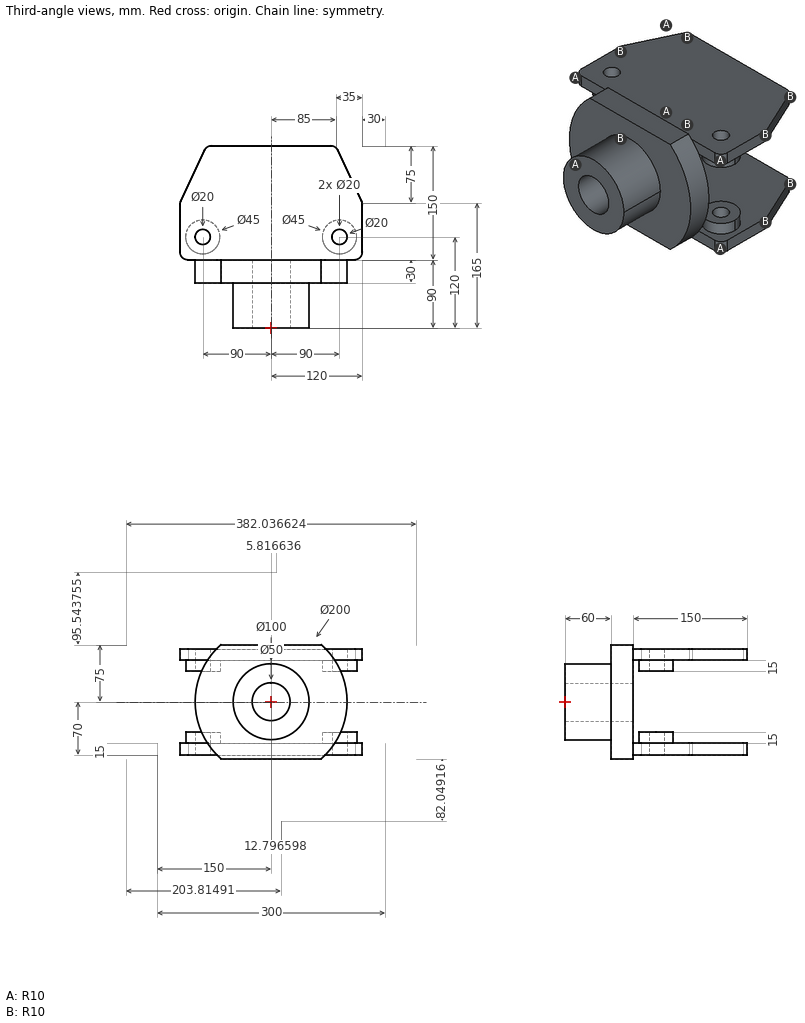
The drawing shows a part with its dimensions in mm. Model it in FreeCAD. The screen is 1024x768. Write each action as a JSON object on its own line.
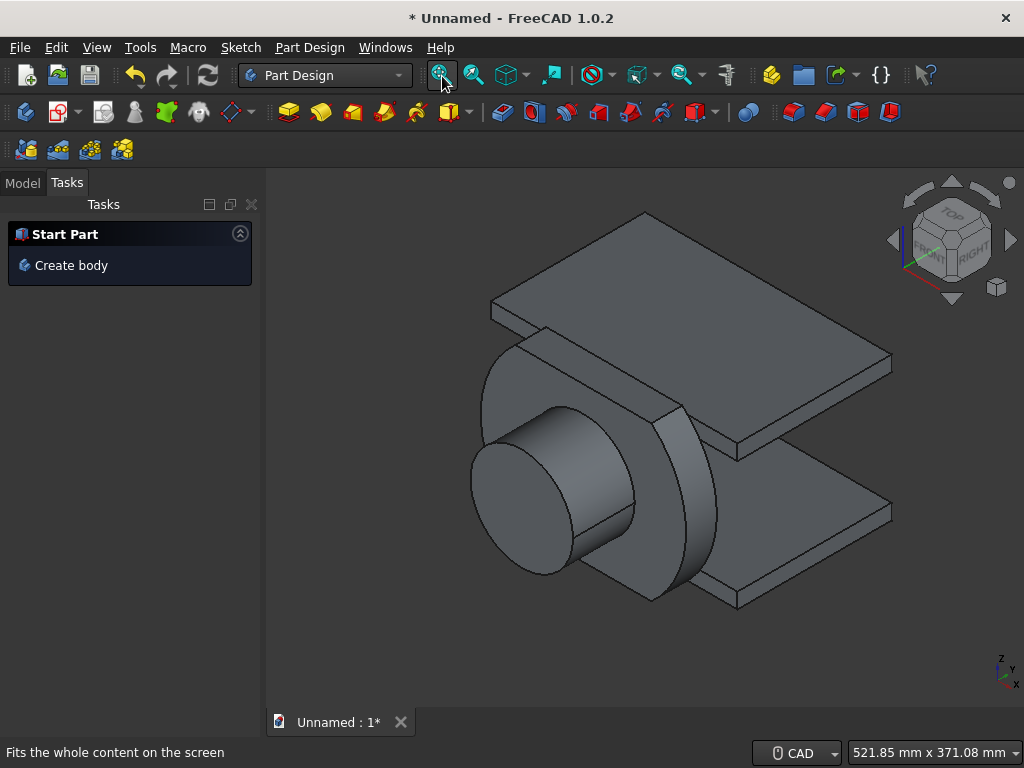
{"action": "left_click", "coordinate": [737, 600]}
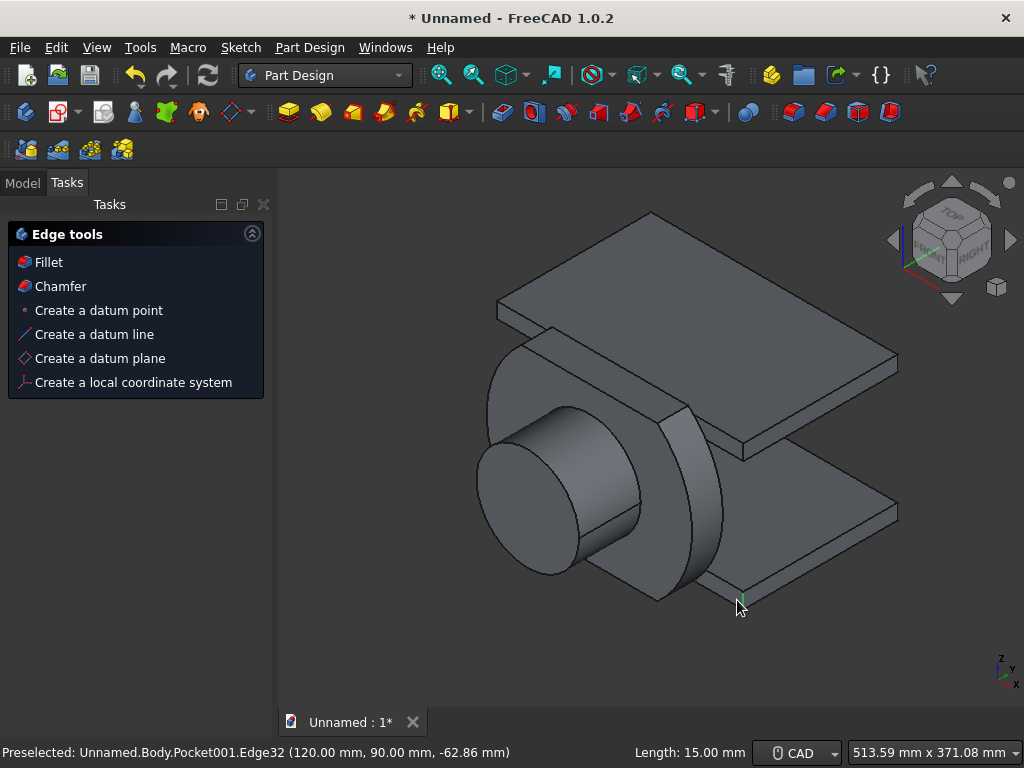
{"action": "left_click", "coordinate": [743, 451], "text": "ctrl"}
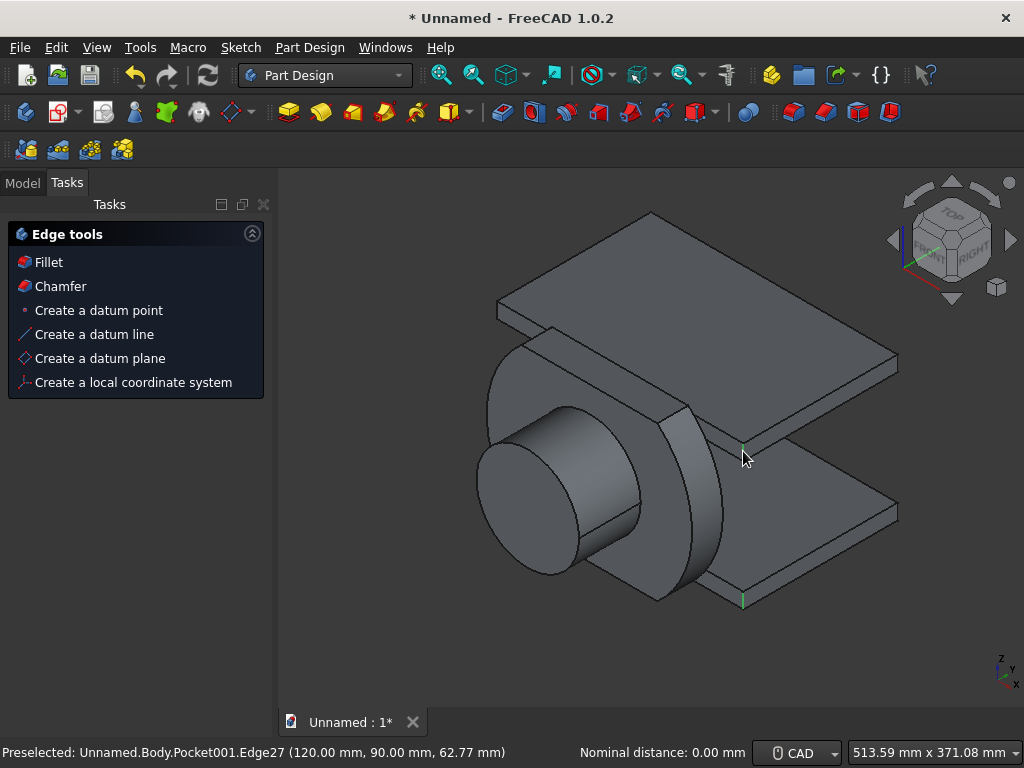
{"action": "scroll", "coordinate": [651, 368], "scroll_direction": "up", "scroll_amount": 4}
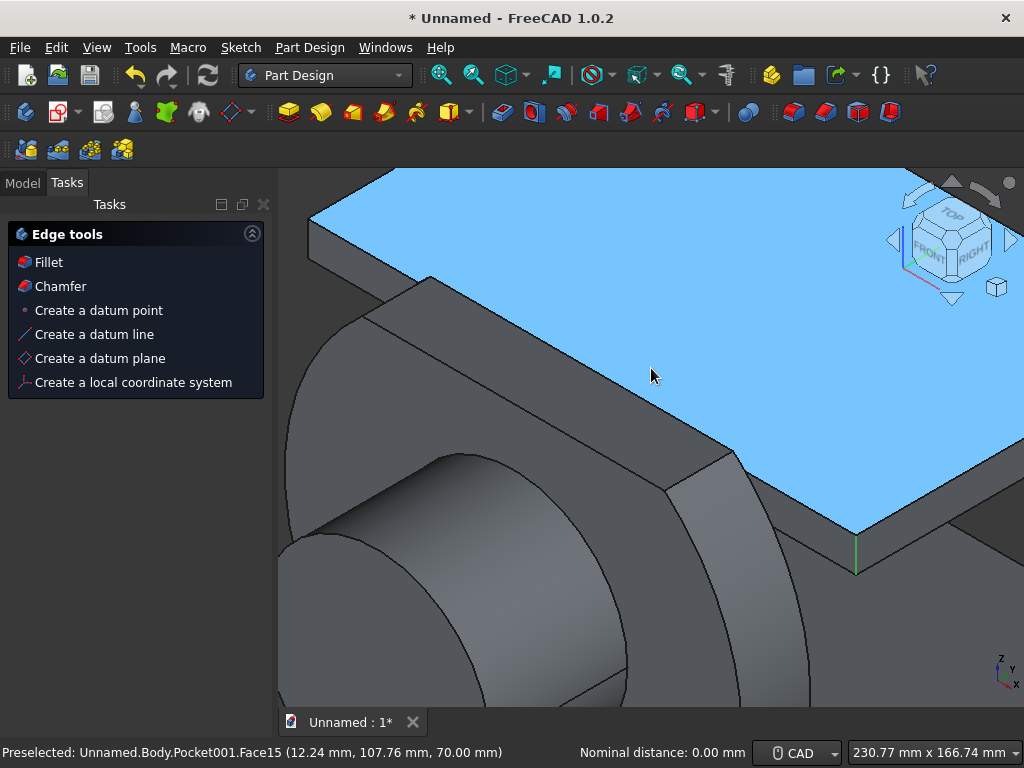
{"action": "key", "text": "v f"}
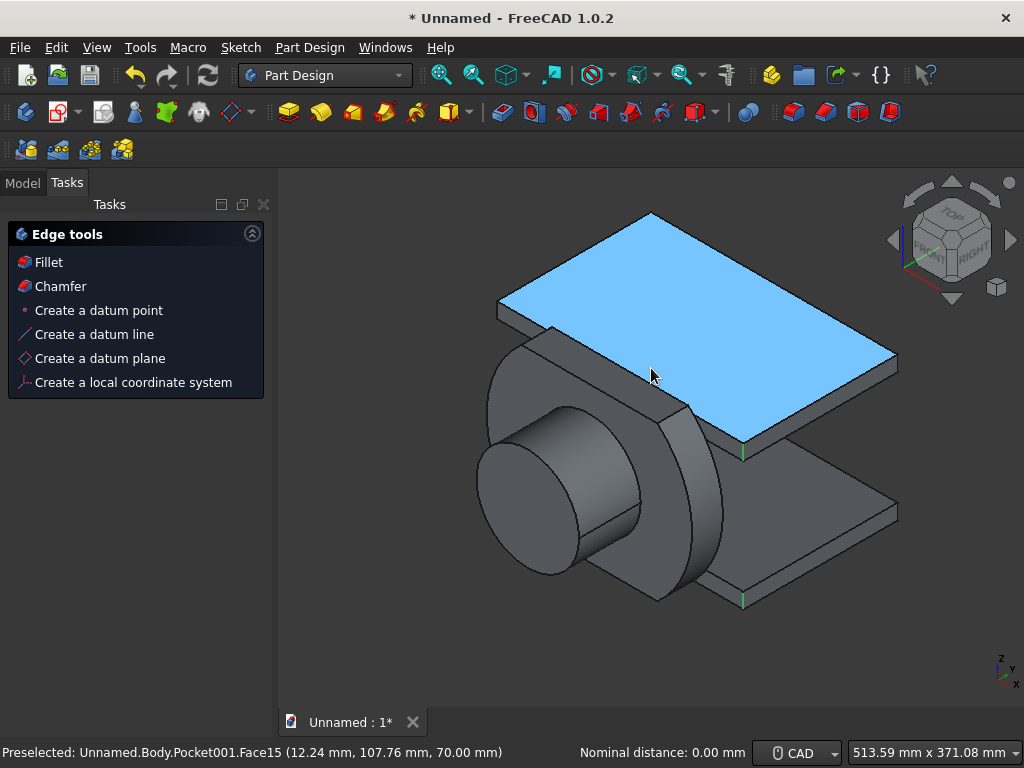
{"action": "key", "text": "2"}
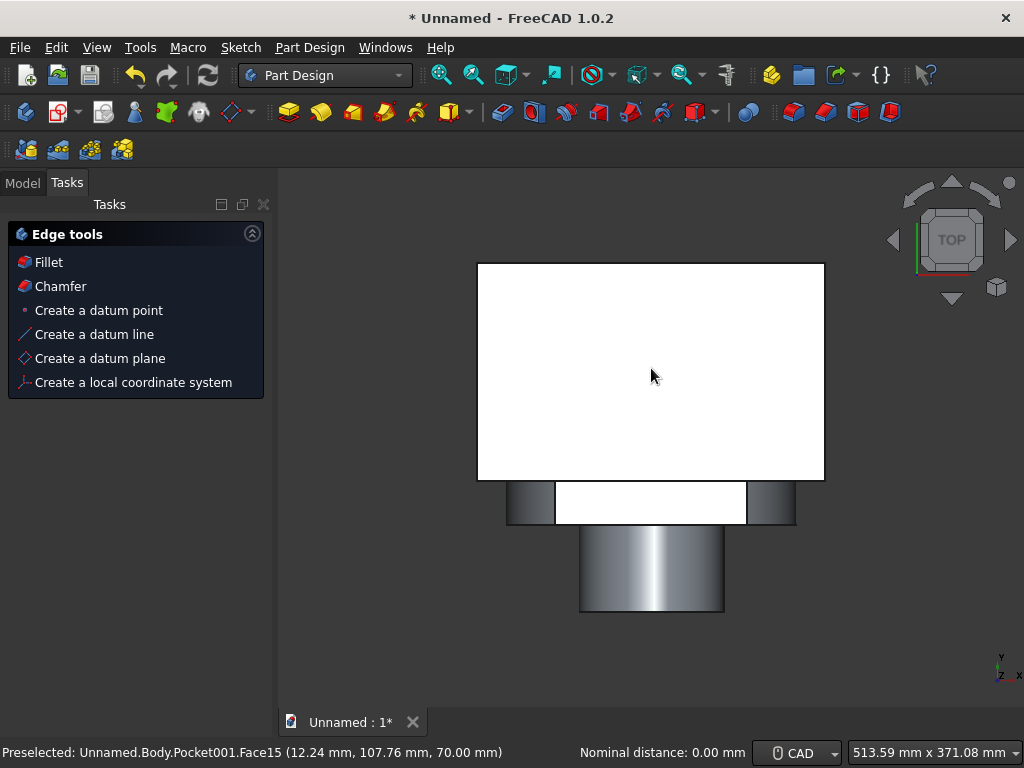
{"action": "scroll", "coordinate": [477, 262], "scroll_direction": "up", "scroll_amount": 4}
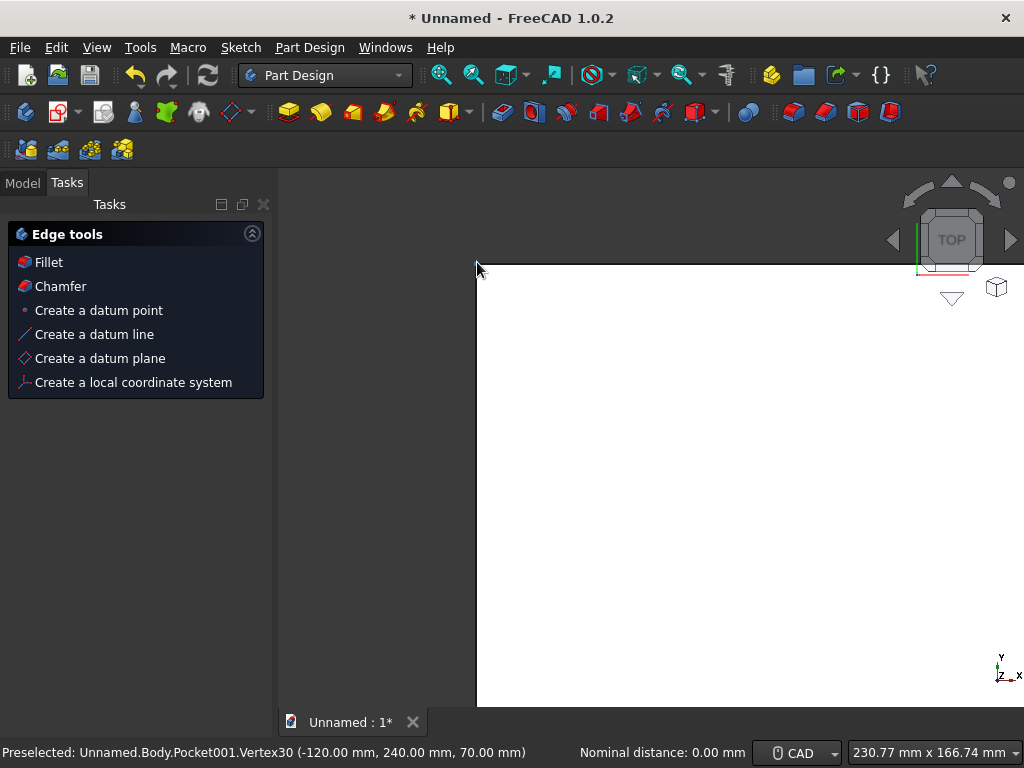
{"action": "key", "text": "v f"}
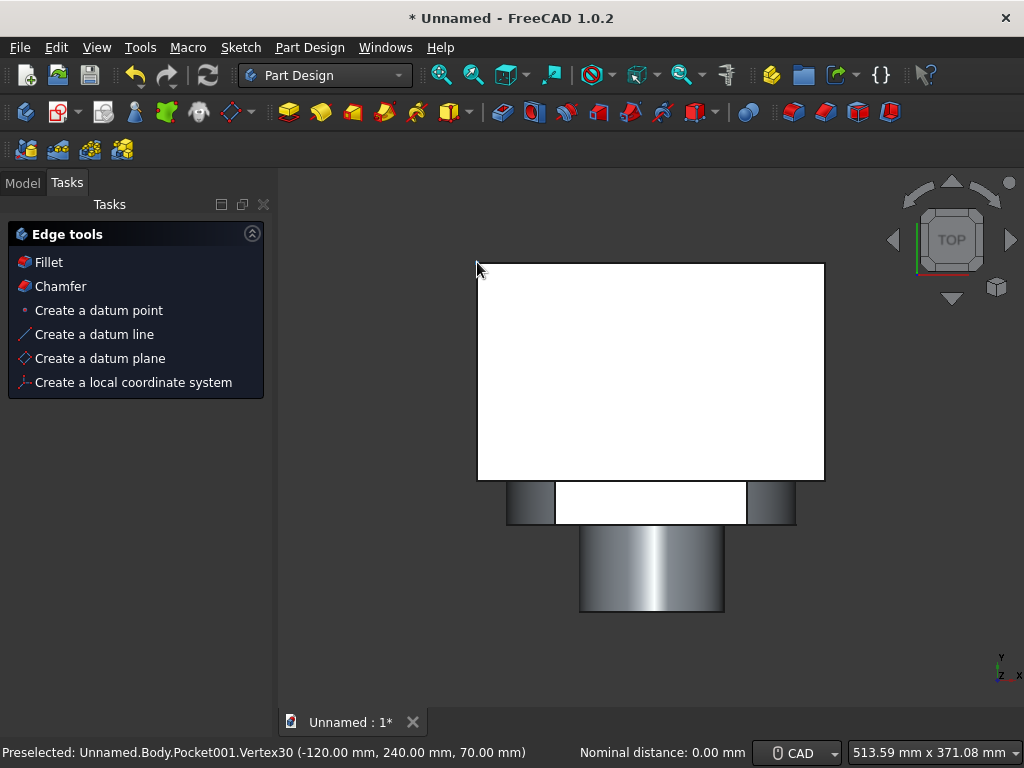
{"action": "key", "text": "1"}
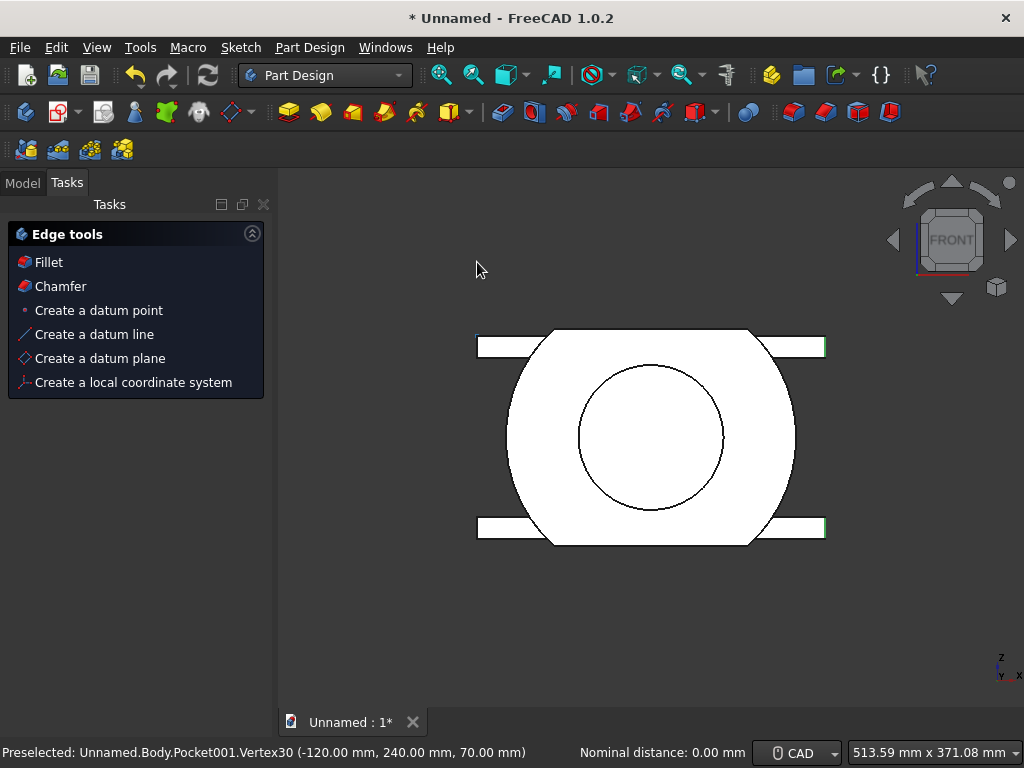
{"action": "left_click", "coordinate": [477, 527], "text": "ctrl"}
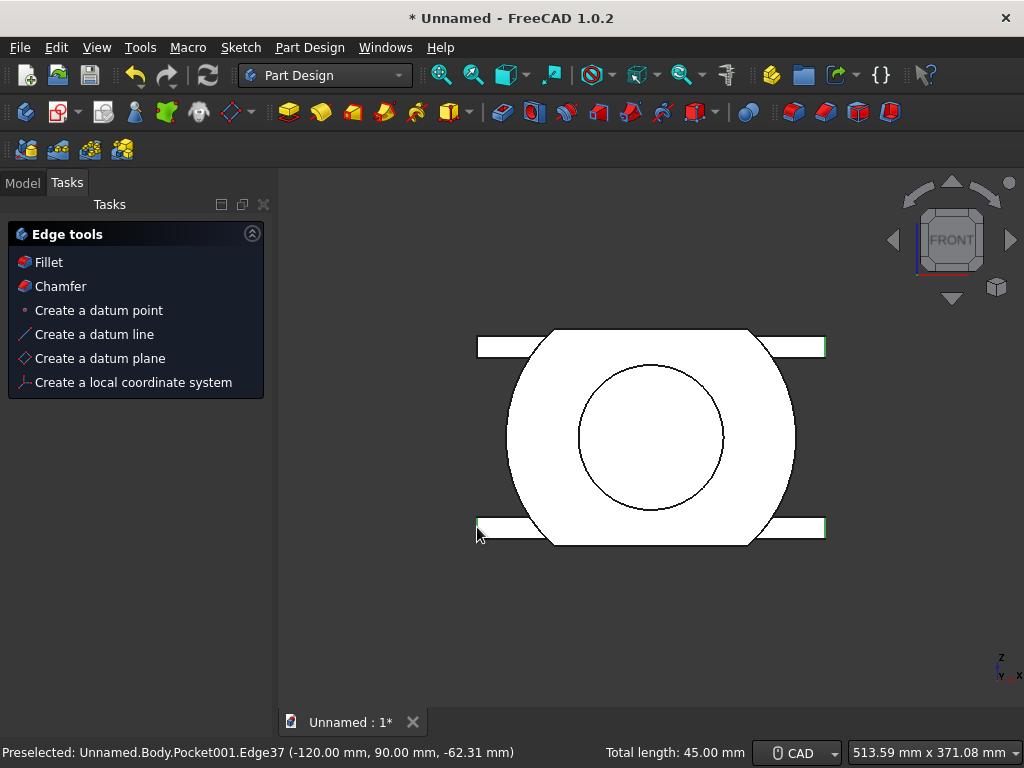
{"action": "left_click", "coordinate": [477, 346], "text": "ctrl"}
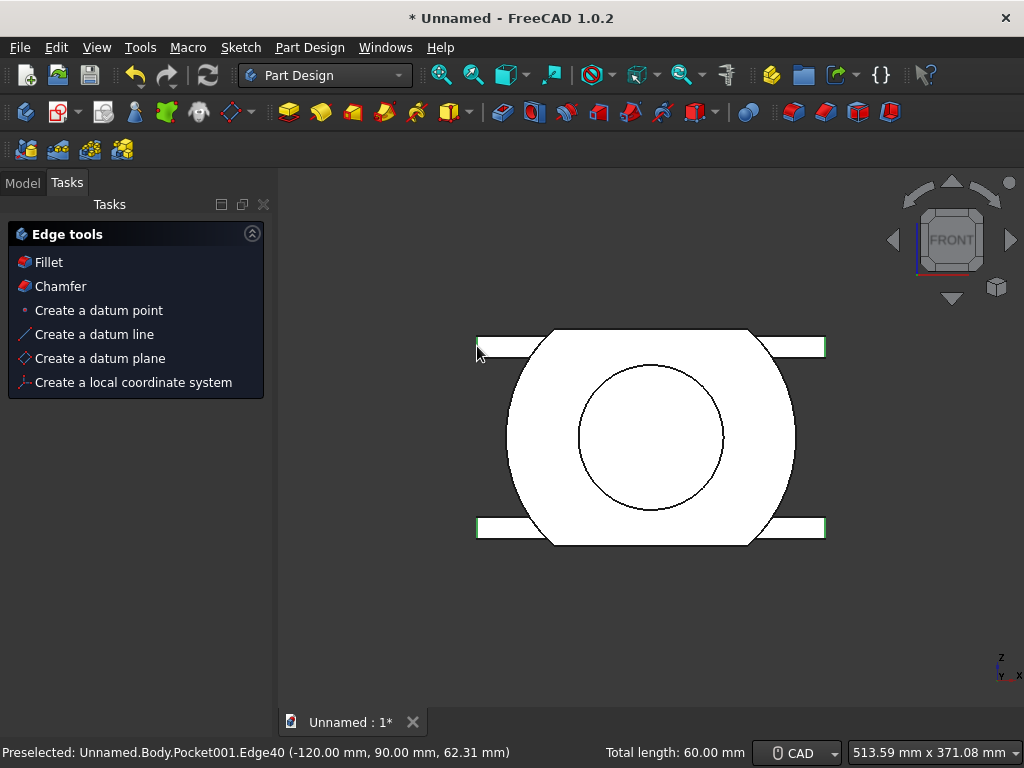
{"action": "scroll", "coordinate": [477, 527], "scroll_direction": "up", "scroll_amount": 4}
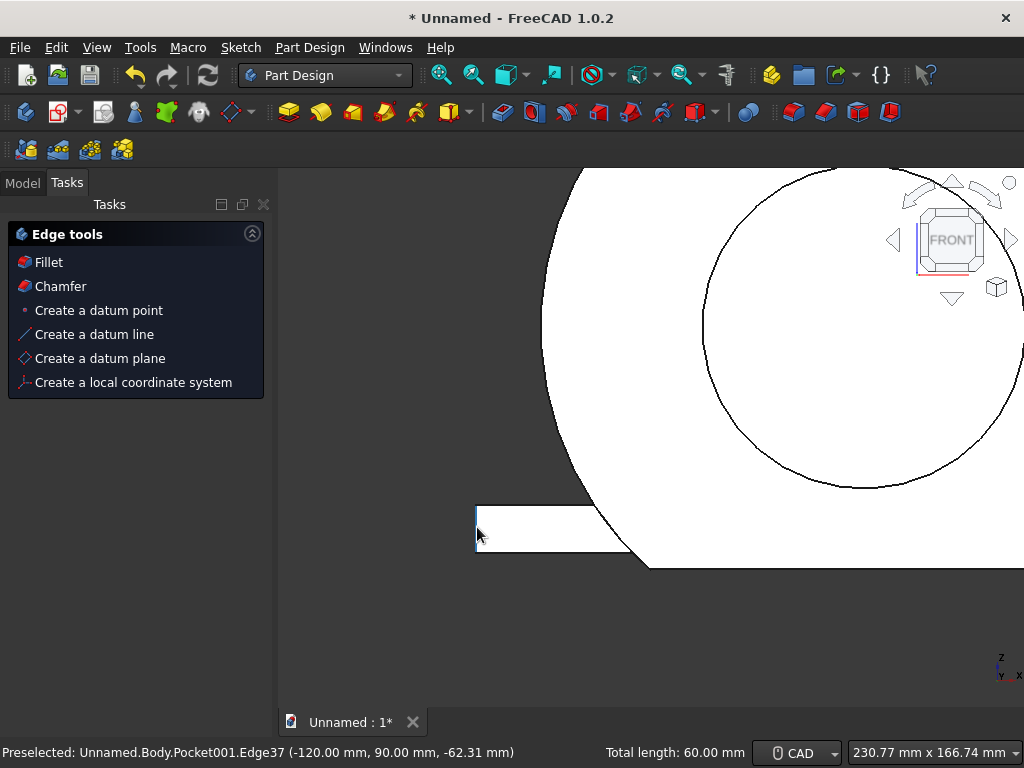
{"action": "left_click", "coordinate": [442, 76]}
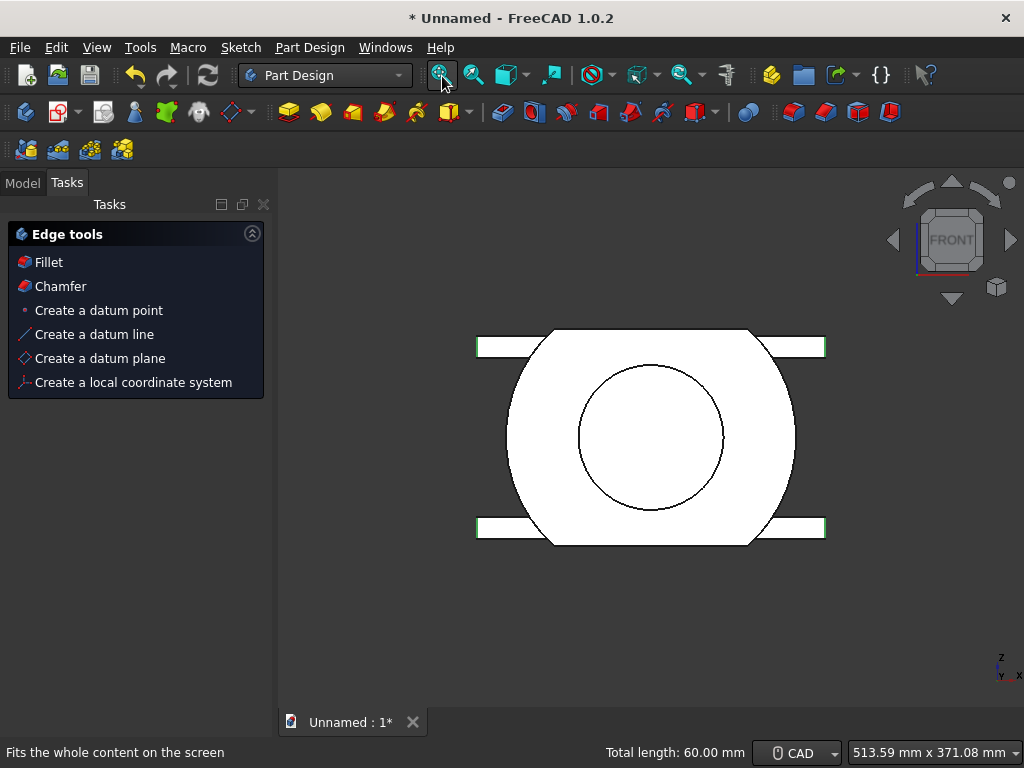
{"action": "key", "text": "3"}